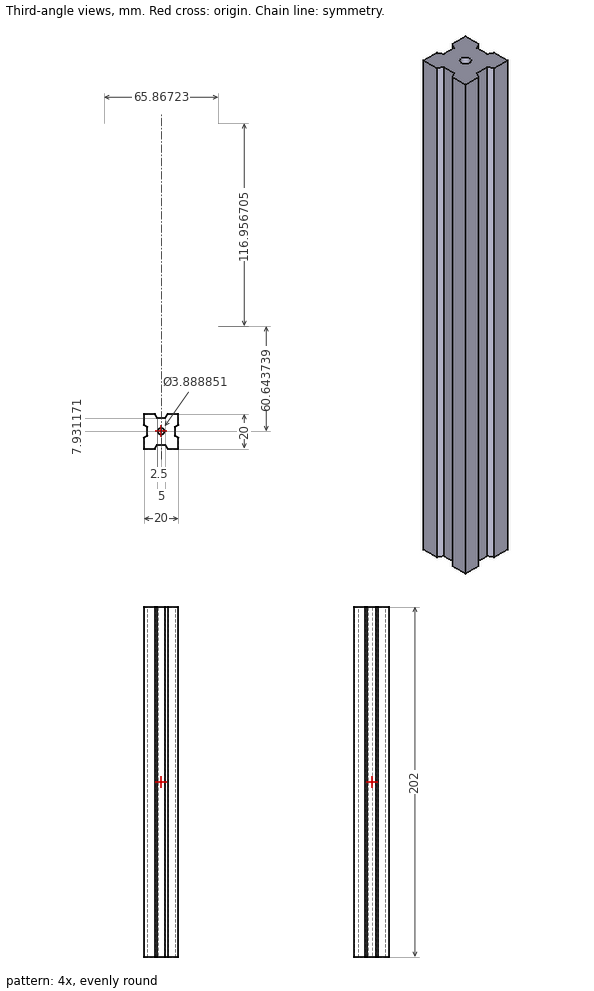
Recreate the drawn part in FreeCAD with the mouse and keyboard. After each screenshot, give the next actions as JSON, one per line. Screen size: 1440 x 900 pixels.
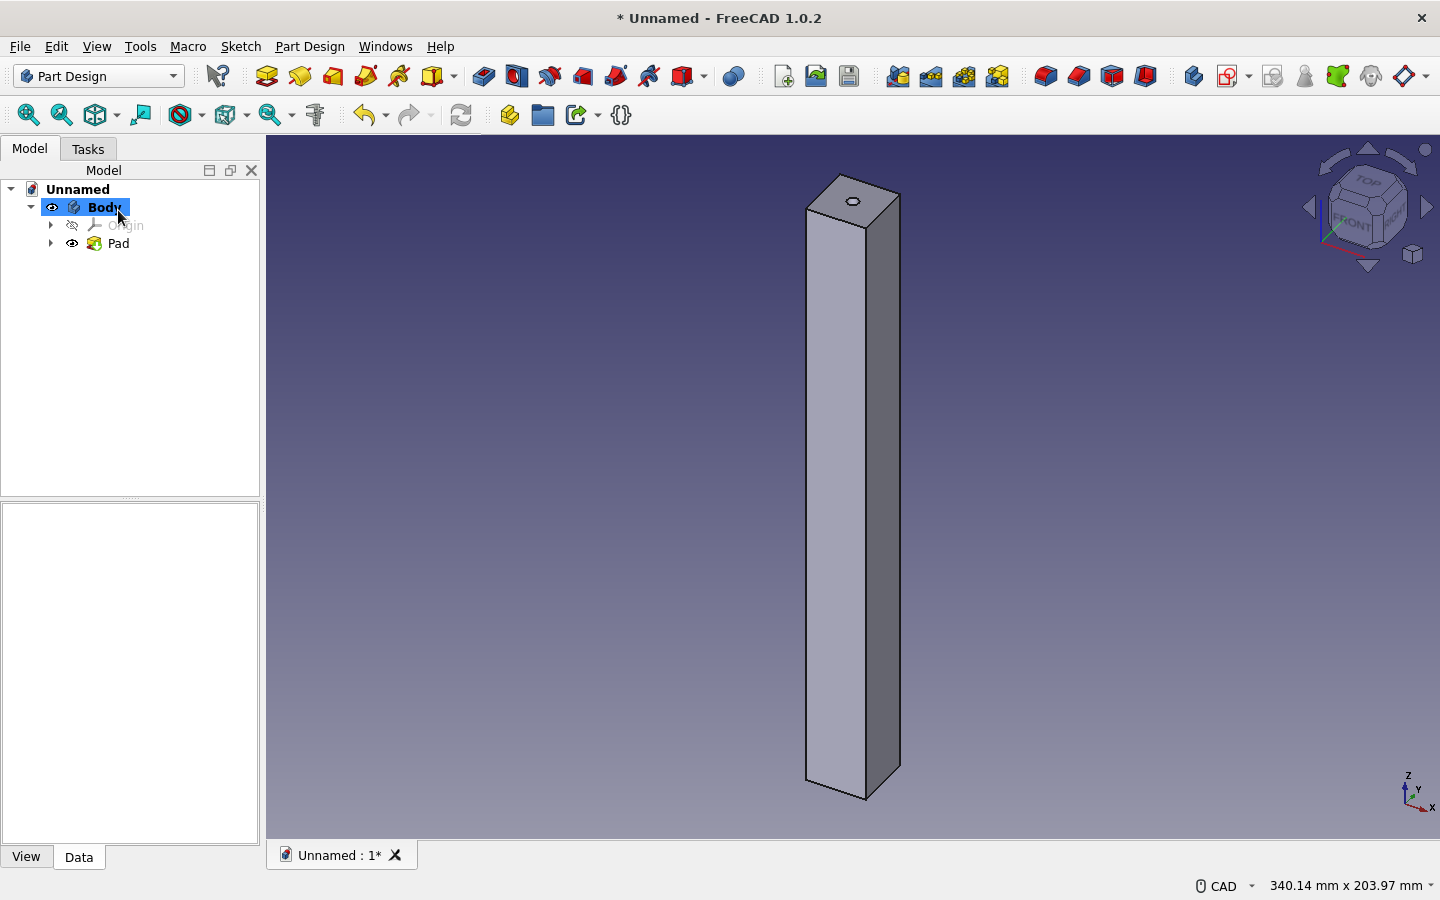
{"action": "left_click", "coordinate": [880, 196]}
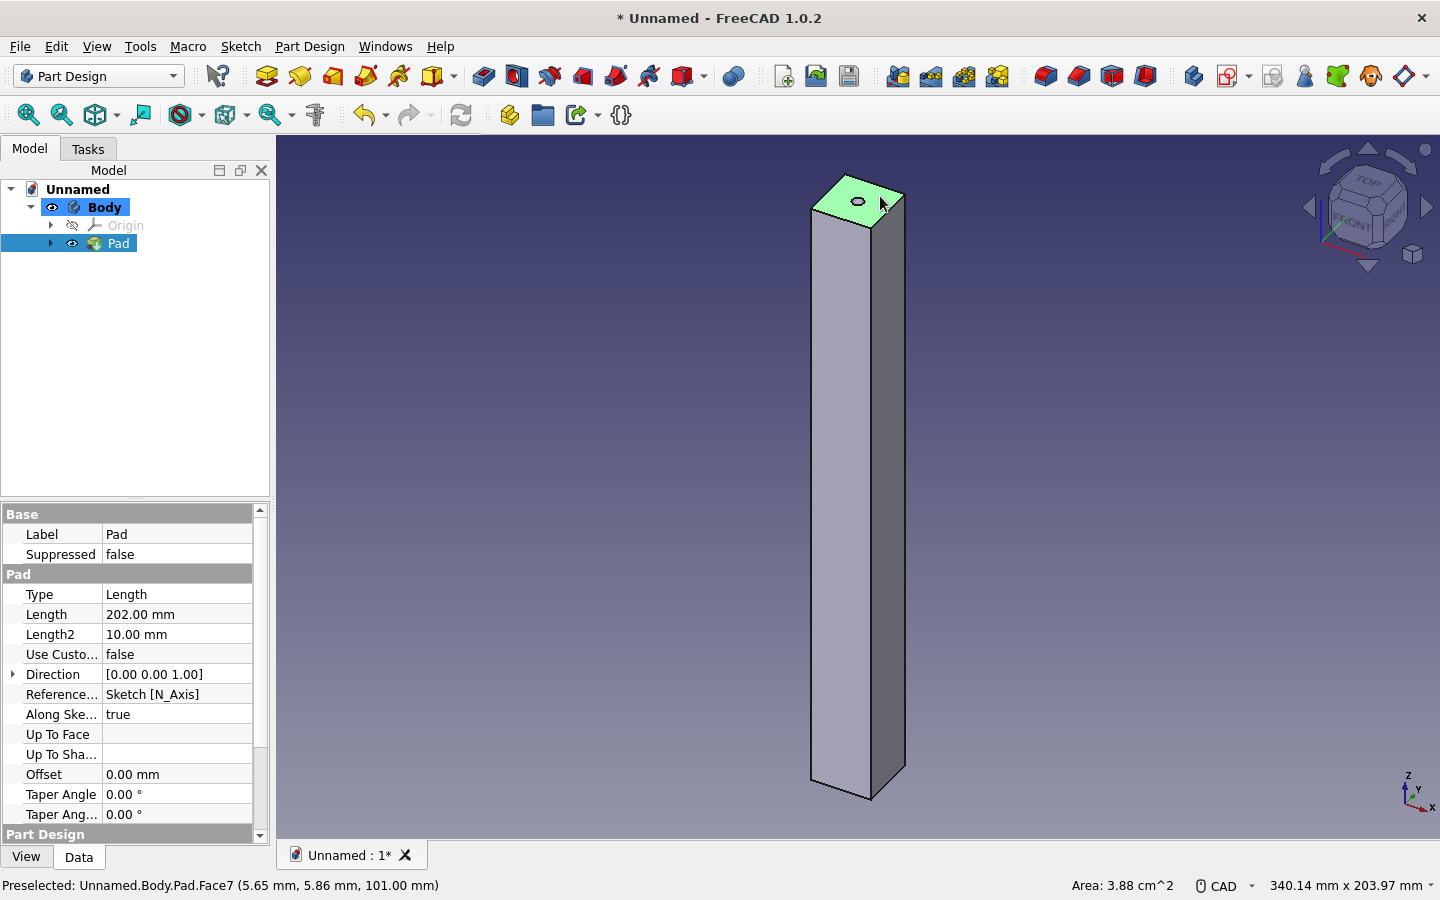
{"action": "left_click", "coordinate": [1226, 76]}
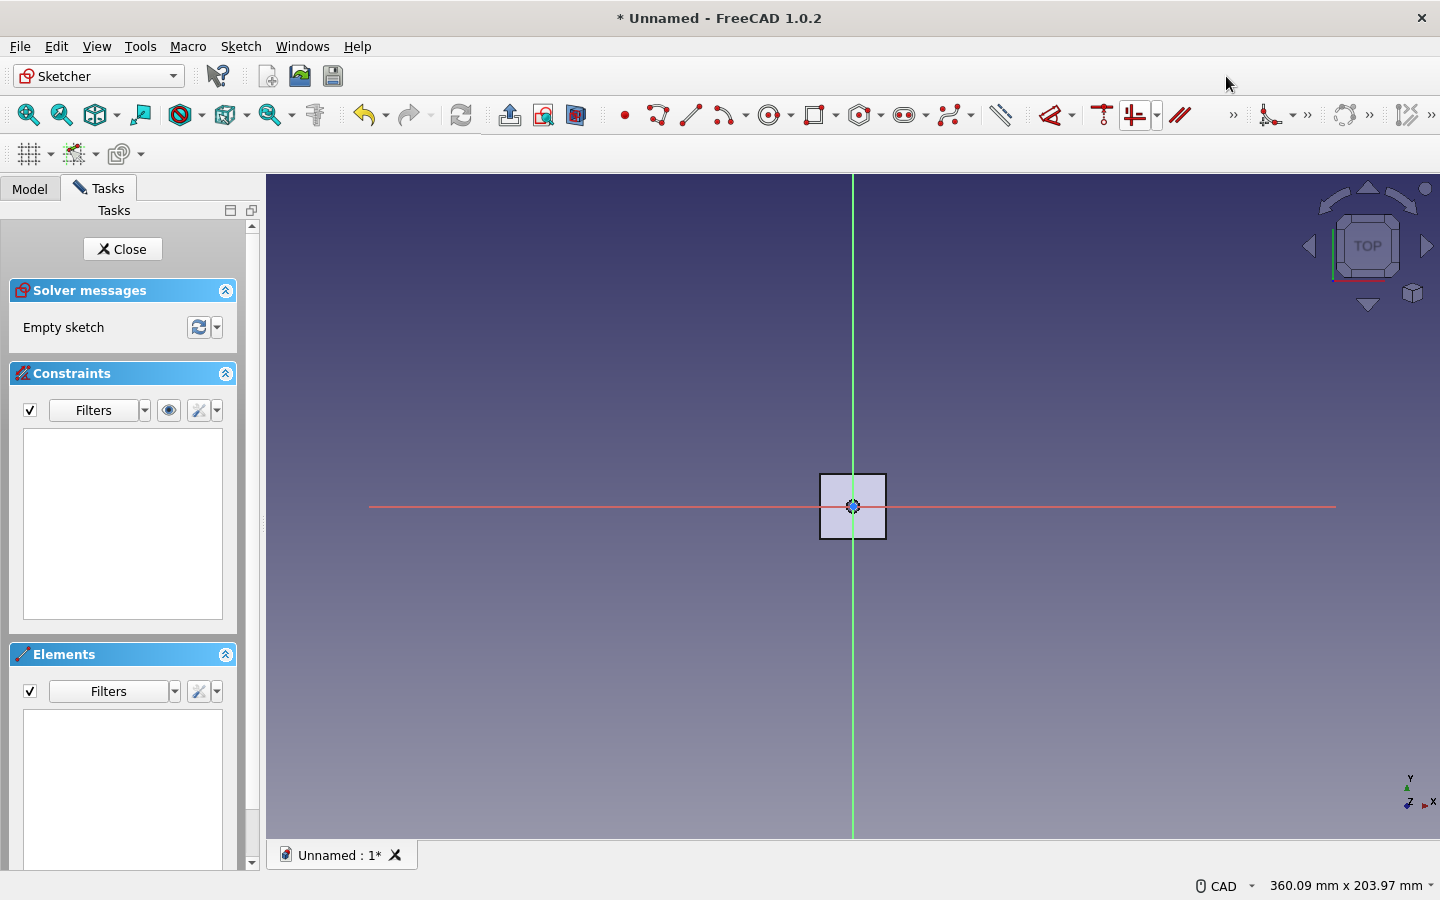
{"action": "scroll", "coordinate": [701, 811], "scroll_direction": "down", "scroll_amount": 3}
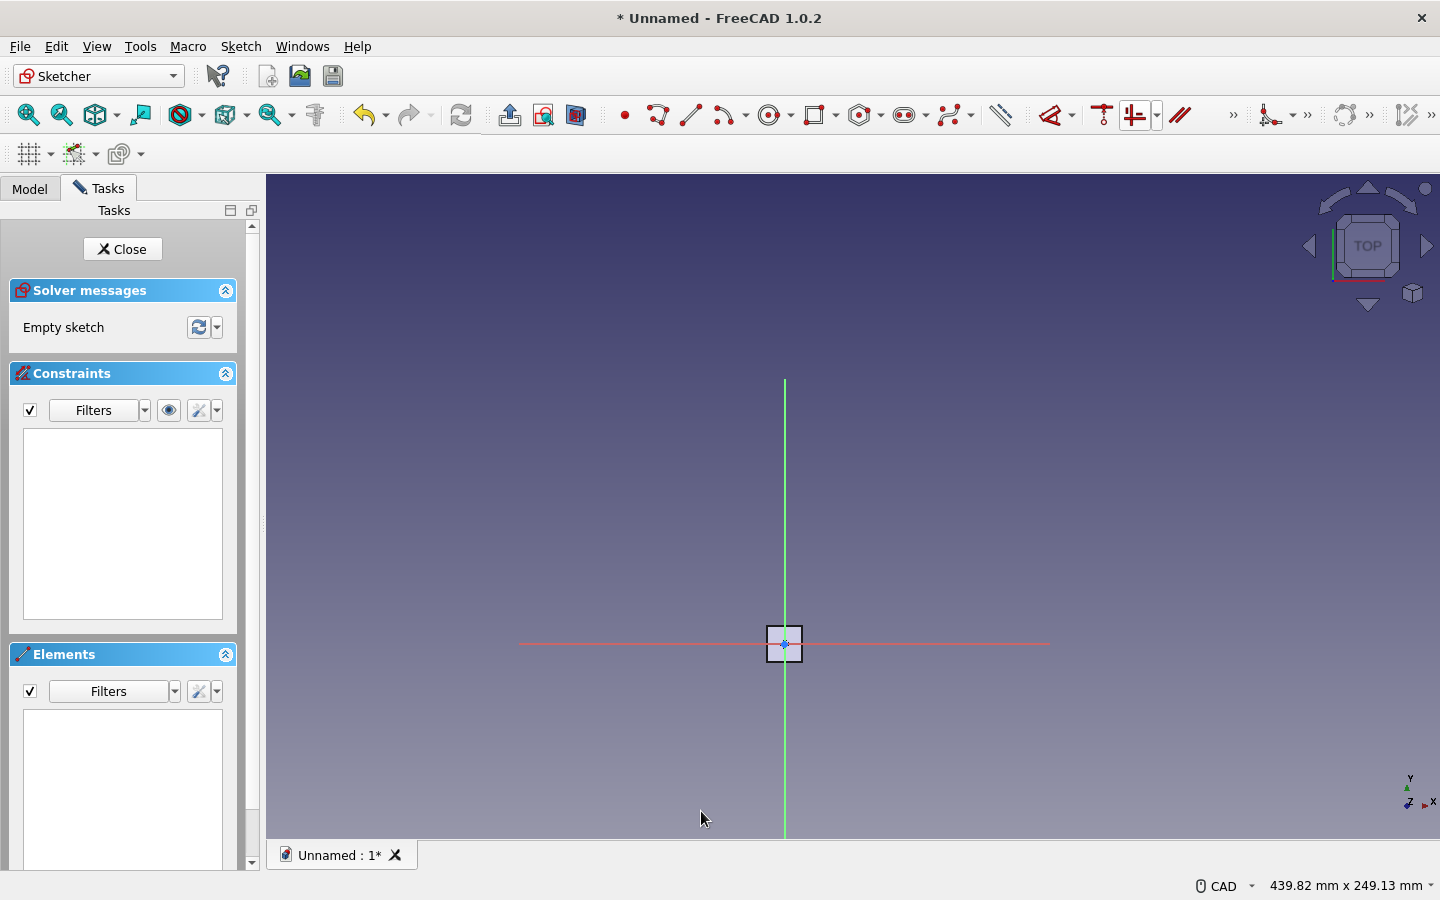
{"action": "scroll", "coordinate": [785, 443], "scroll_direction": "up", "scroll_amount": 2}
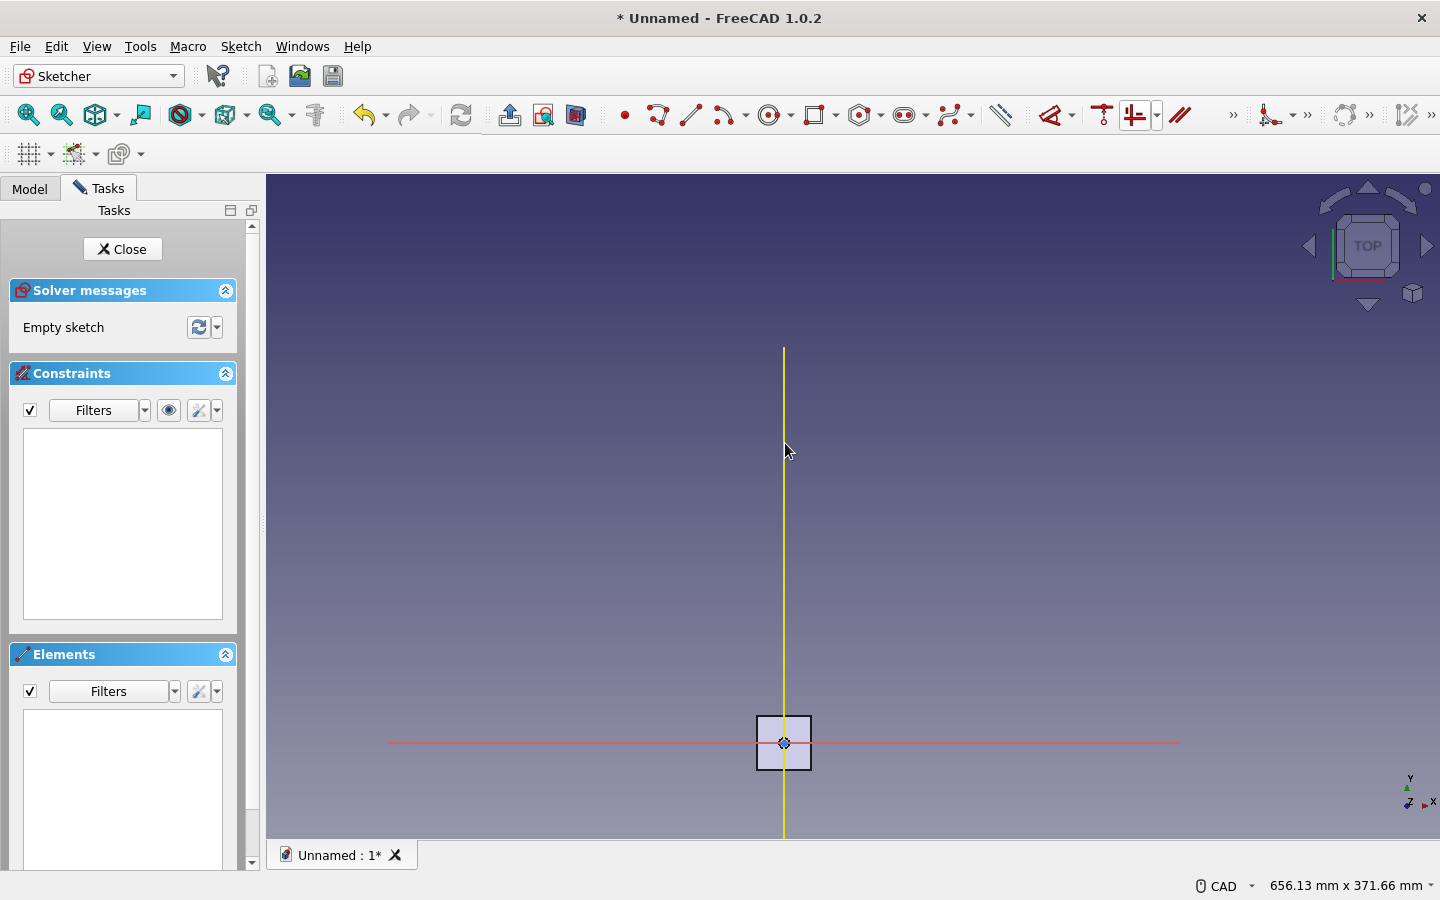
{"action": "left_click", "coordinate": [658, 116]}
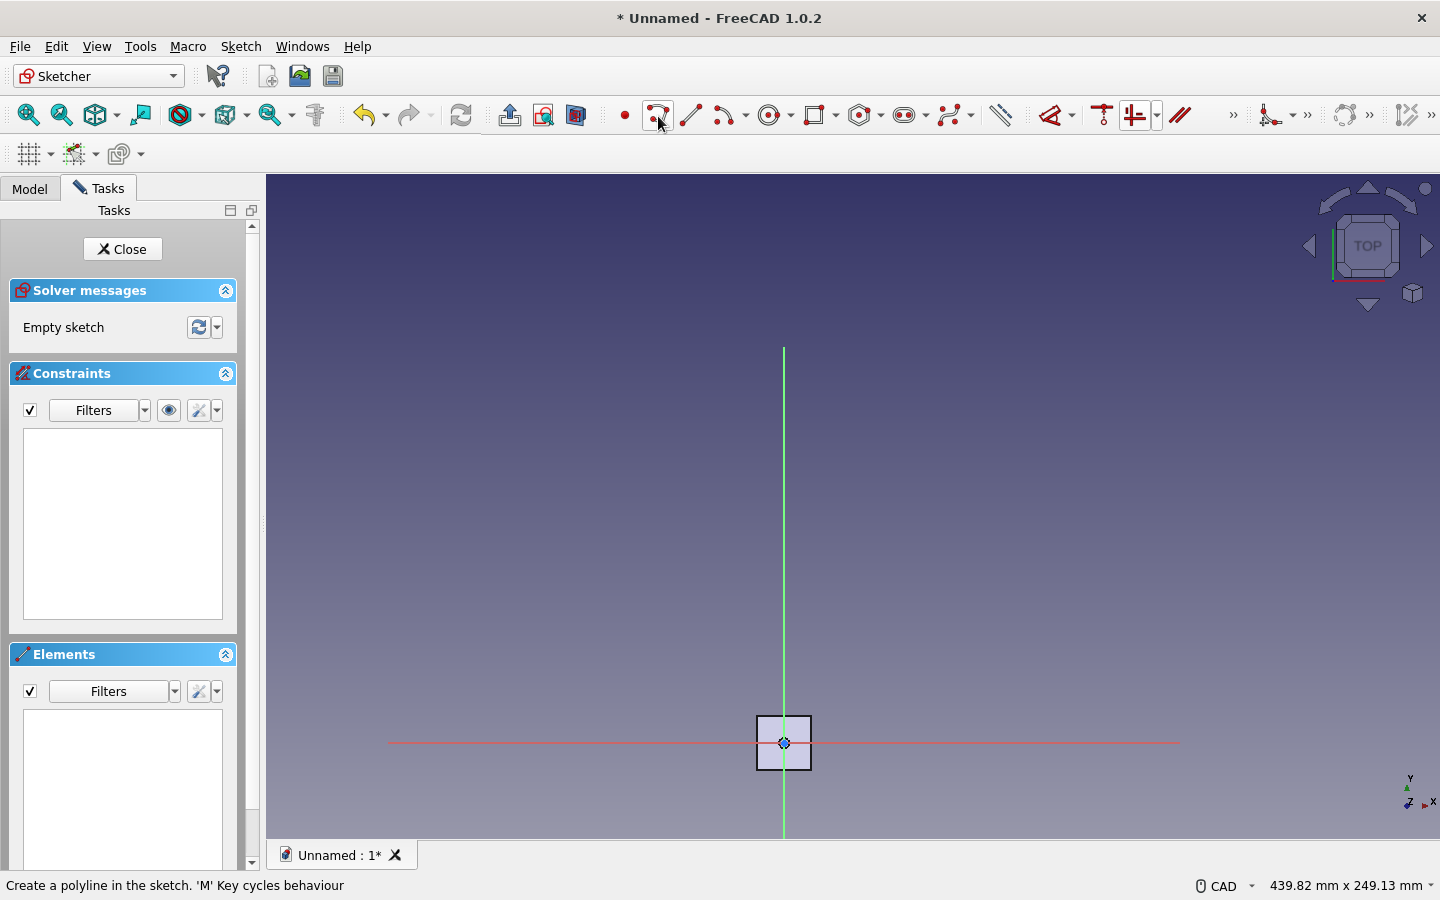
{"action": "scroll", "coordinate": [777, 722], "scroll_direction": "up", "scroll_amount": 5}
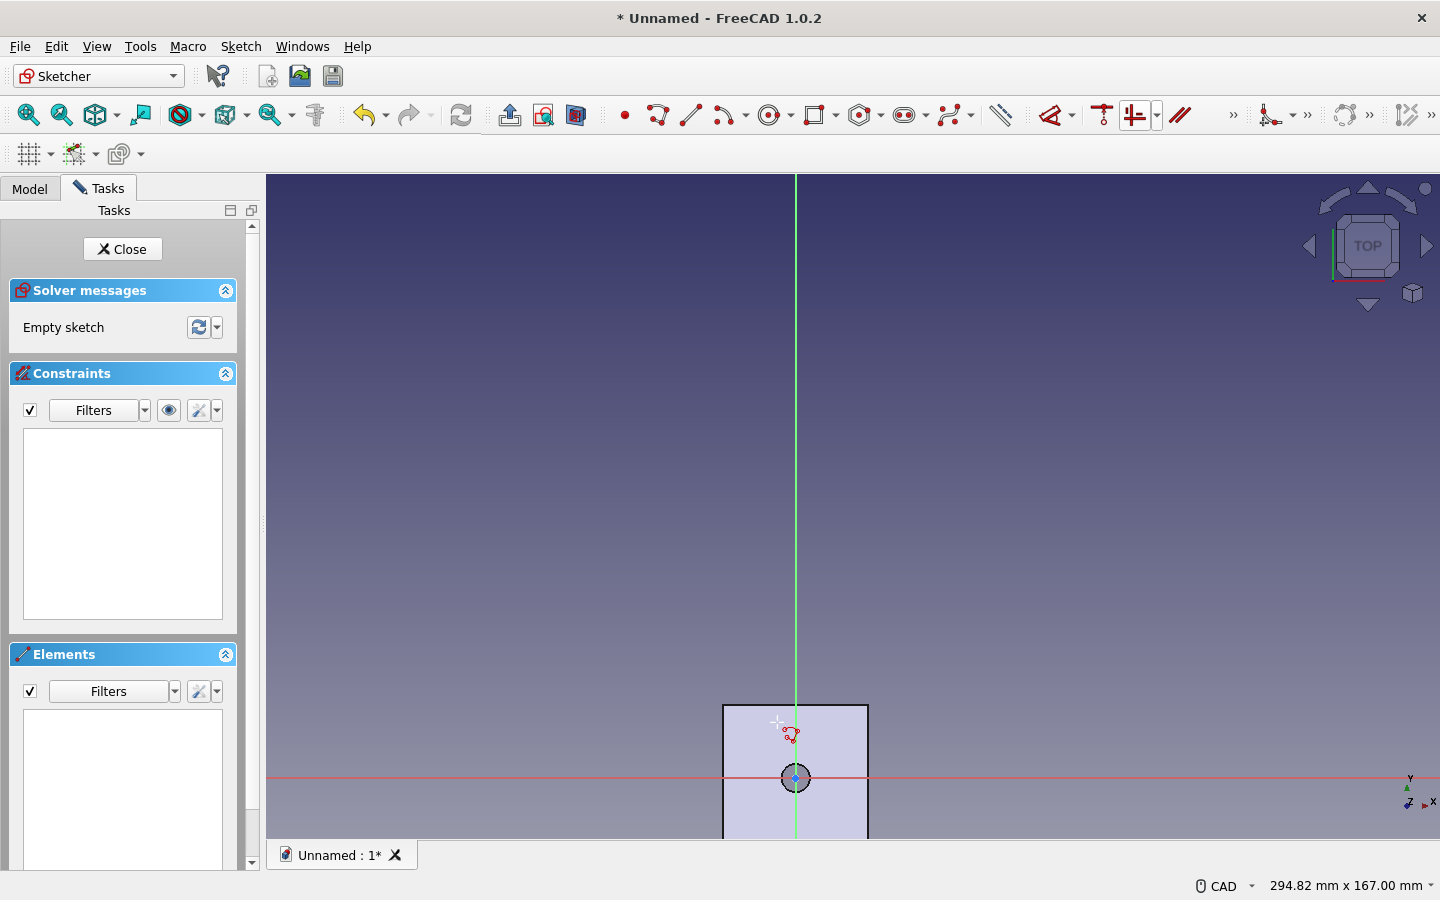
{"action": "left_click", "coordinate": [778, 720]}
{"action": "left_click", "coordinate": [814, 720]}
{"action": "left_click", "coordinate": [1035, 338]}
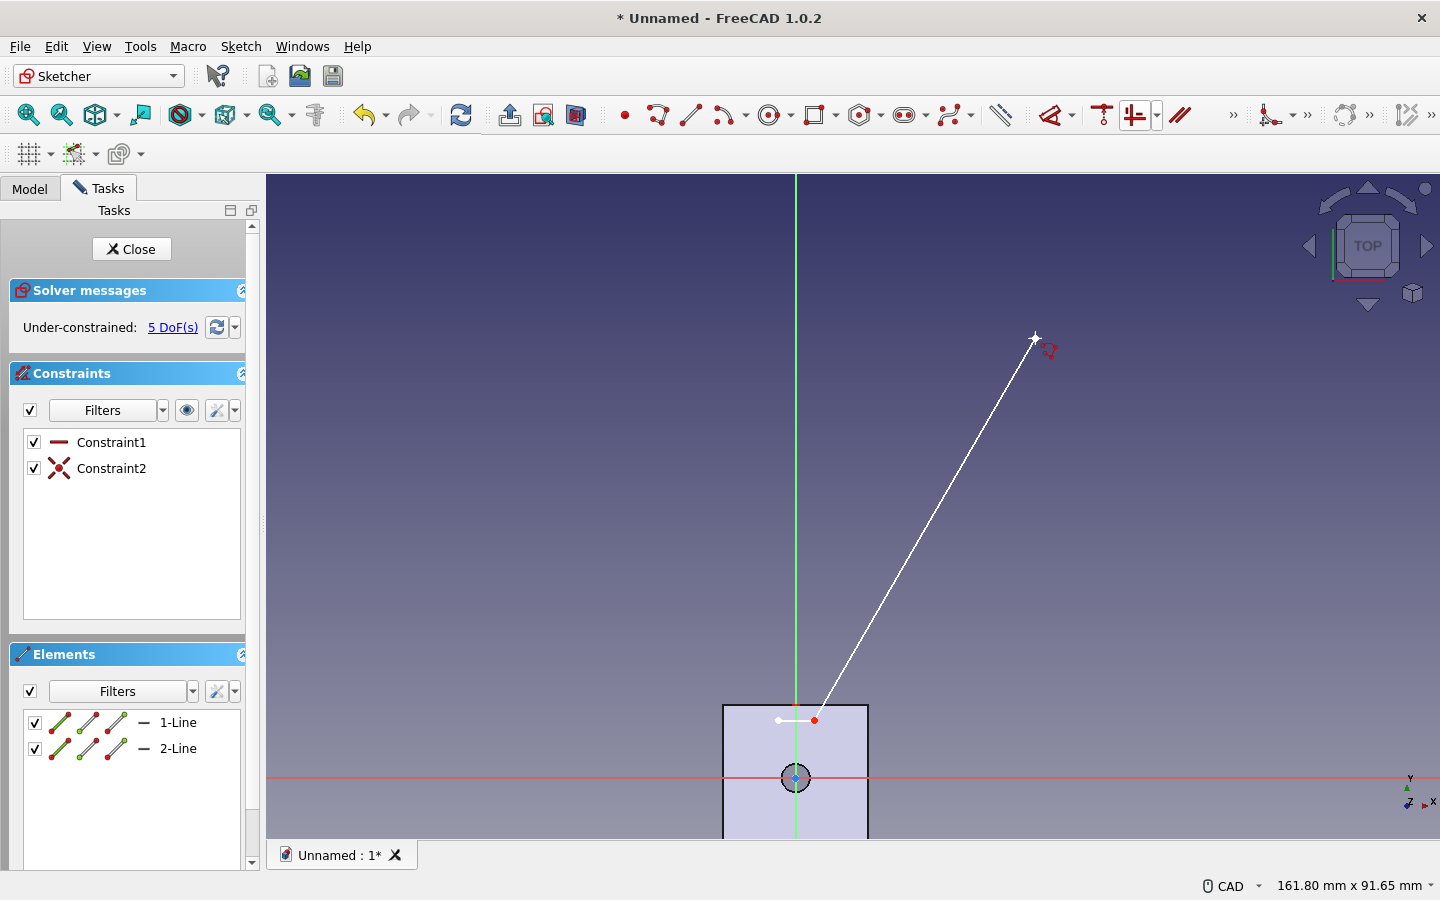
{"action": "scroll", "coordinate": [778, 723], "scroll_direction": "down", "scroll_amount": 5}